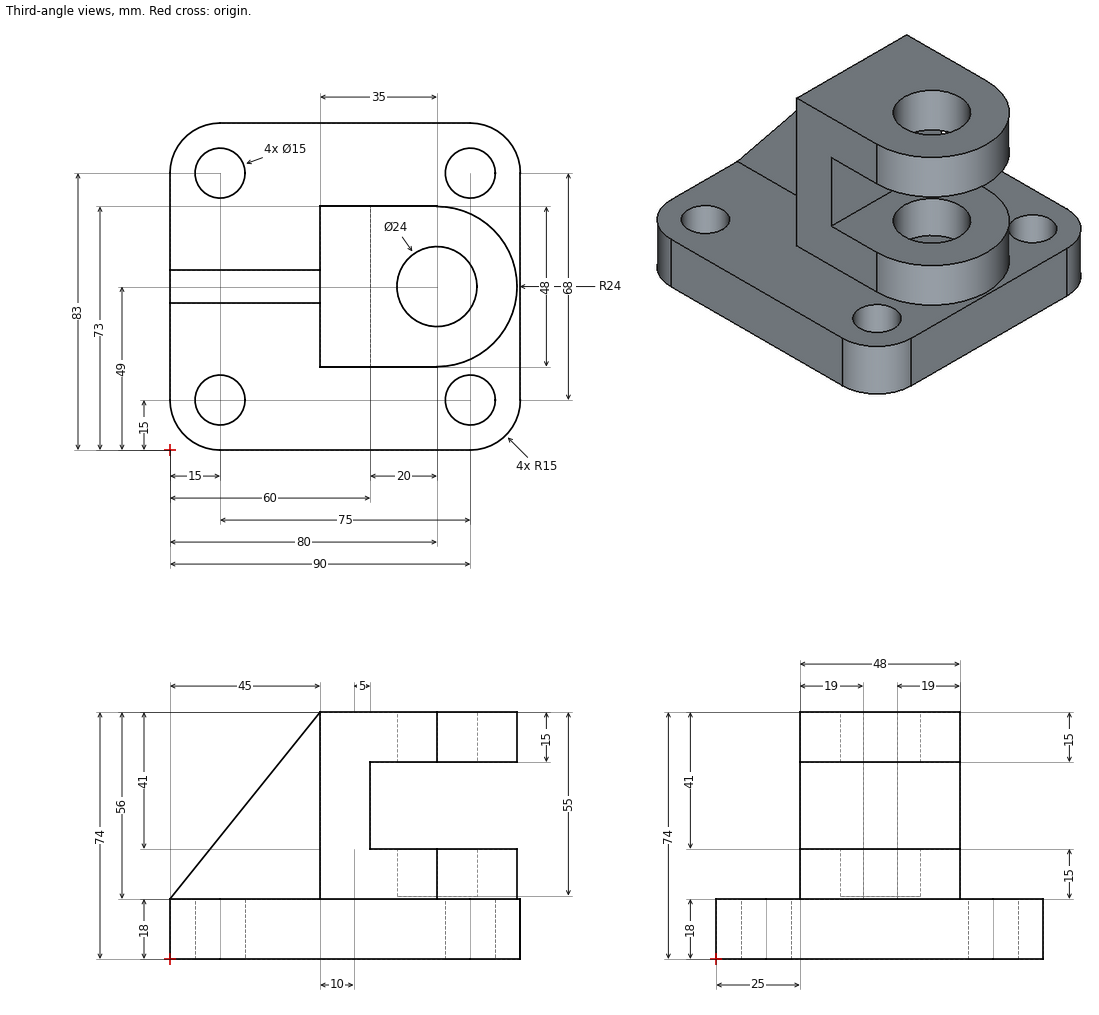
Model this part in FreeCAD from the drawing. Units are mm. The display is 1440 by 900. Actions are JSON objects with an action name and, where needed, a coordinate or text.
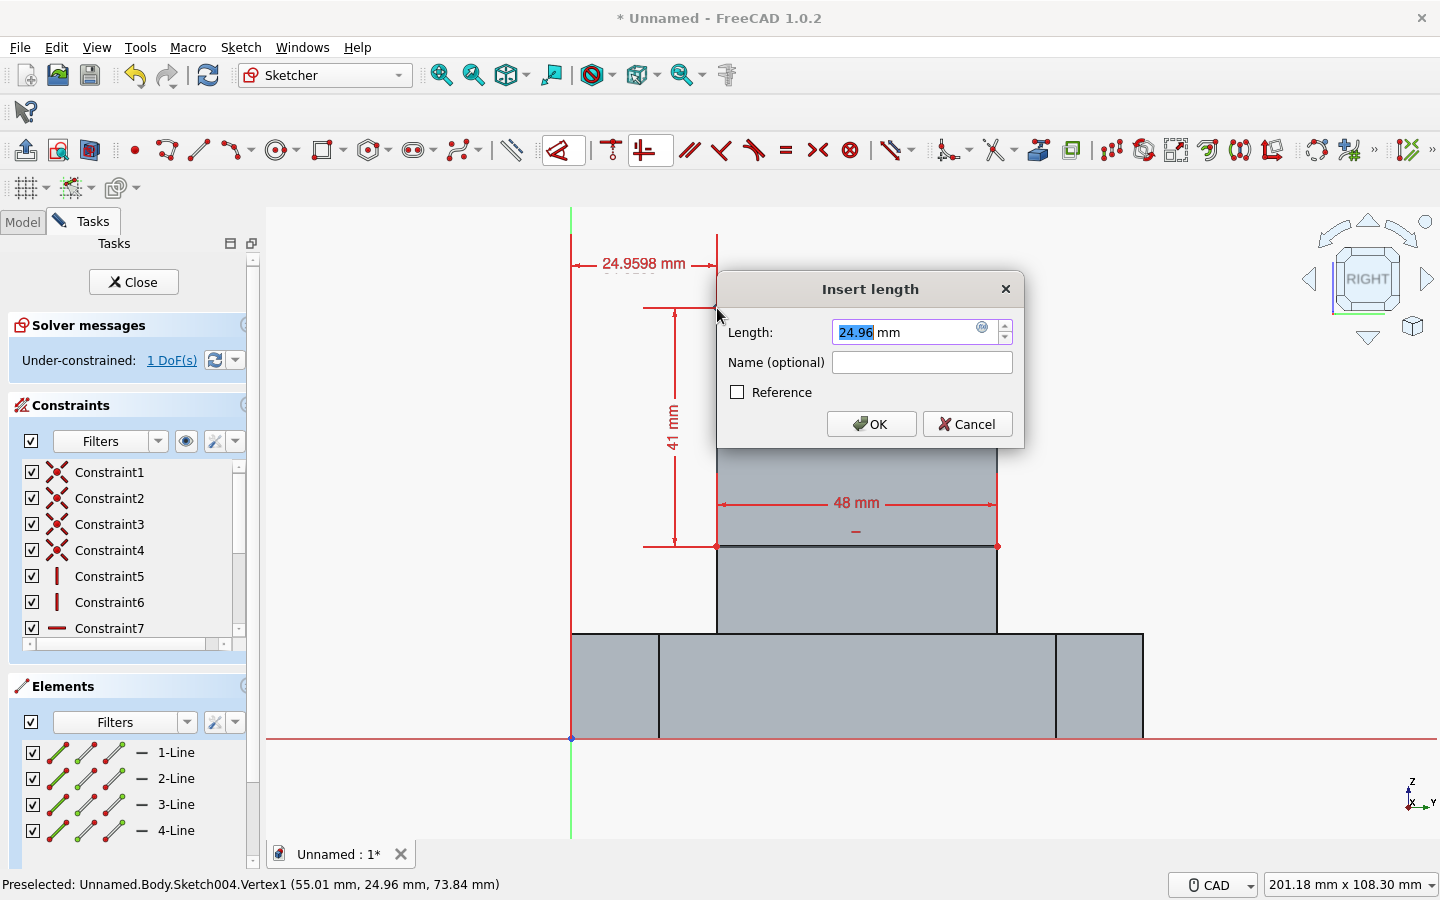
{"action": "type", "text": "25"}
{"action": "key", "text": "Return"}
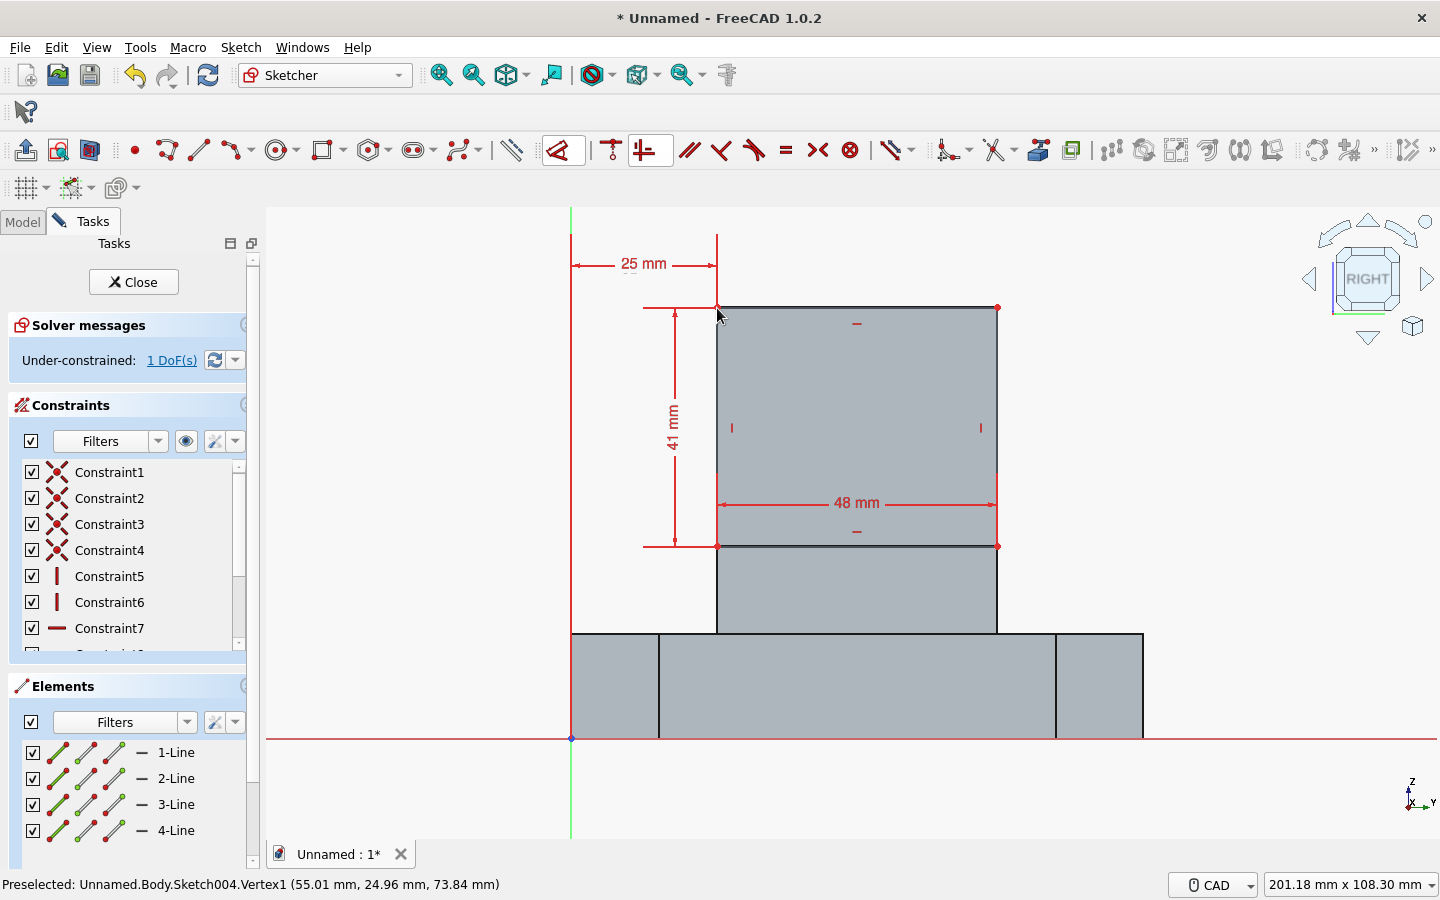
{"action": "left_click", "coordinate": [717, 308]}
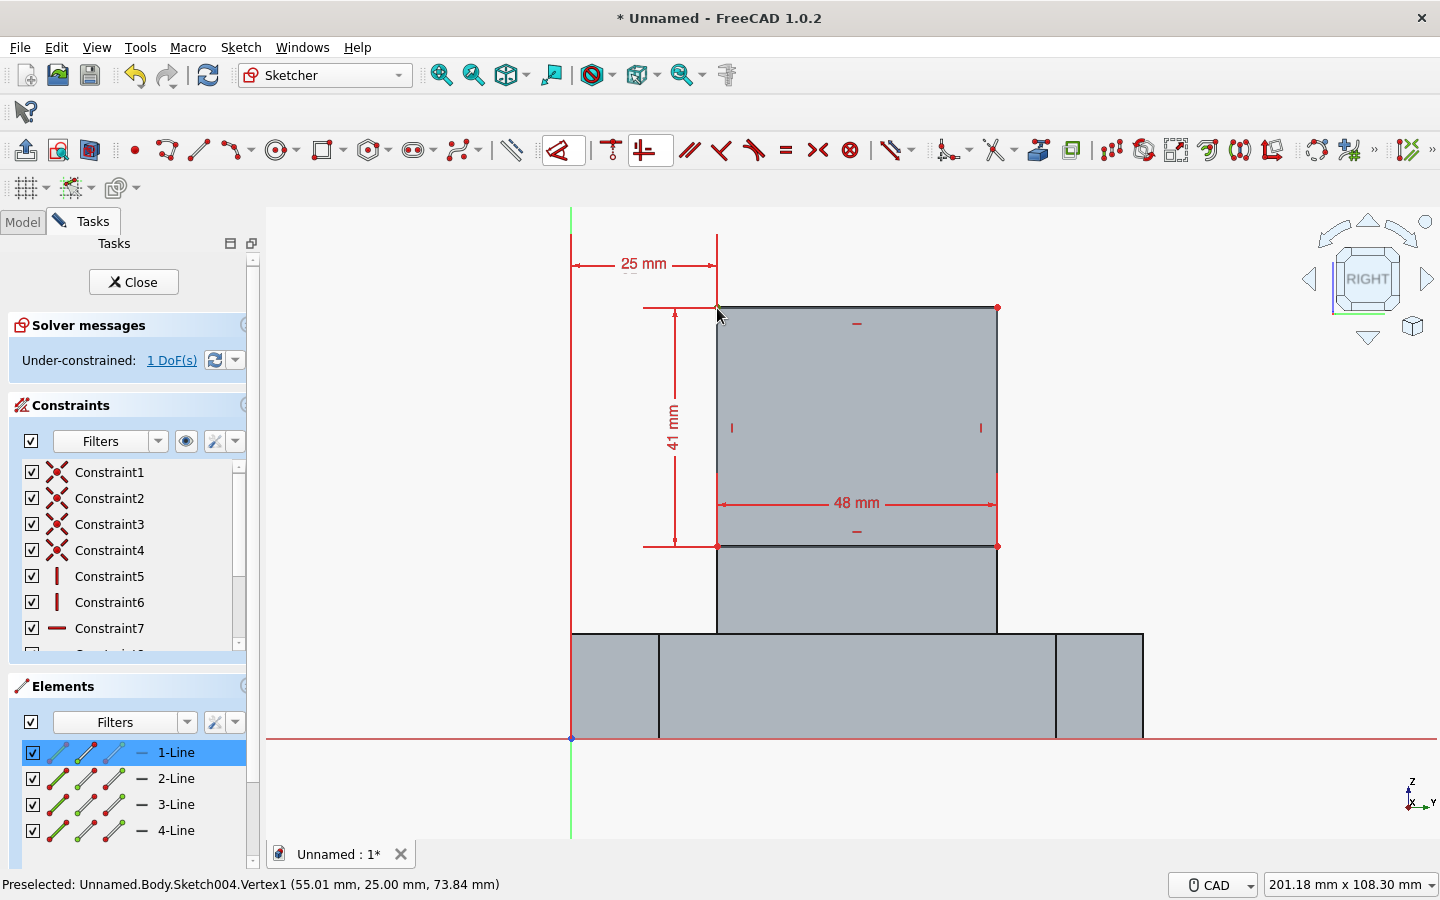
{"action": "left_click", "coordinate": [580, 150]}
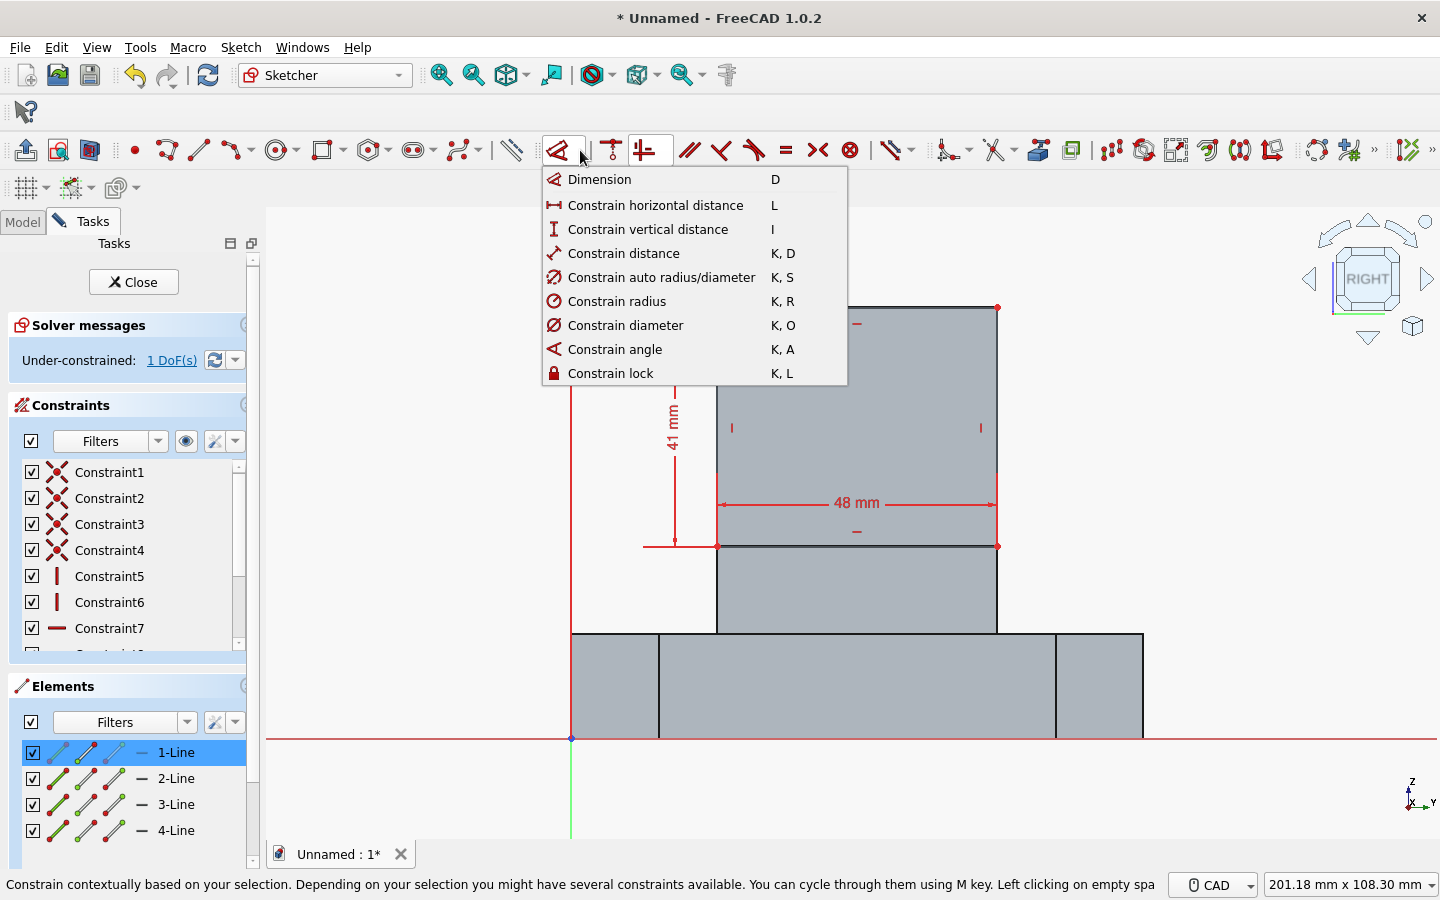
{"action": "left_click", "coordinate": [695, 229]}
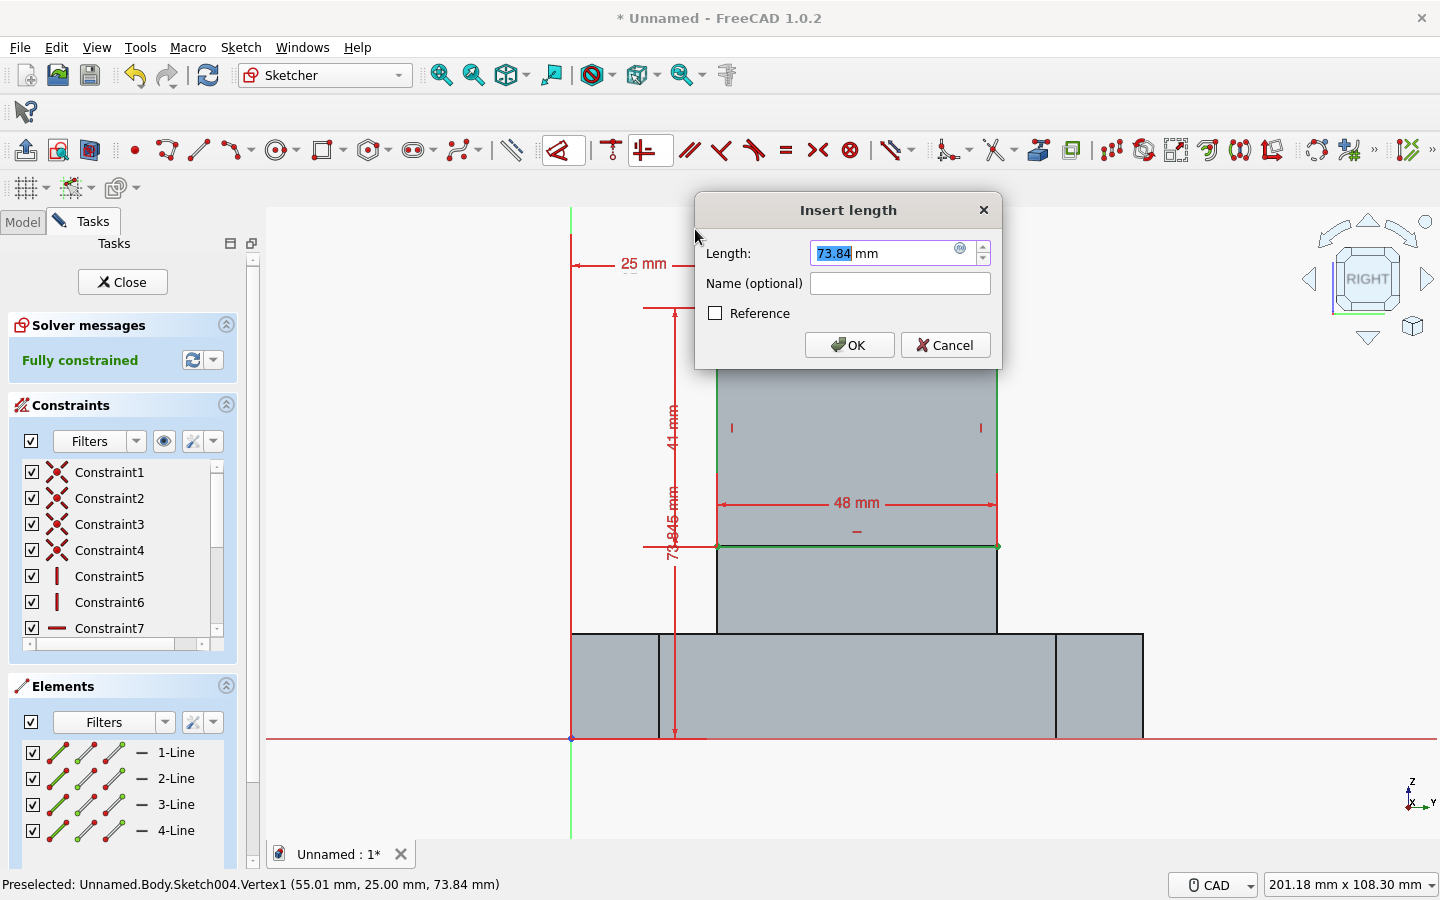
{"action": "type", "text": "74"}
{"action": "key", "text": "Return"}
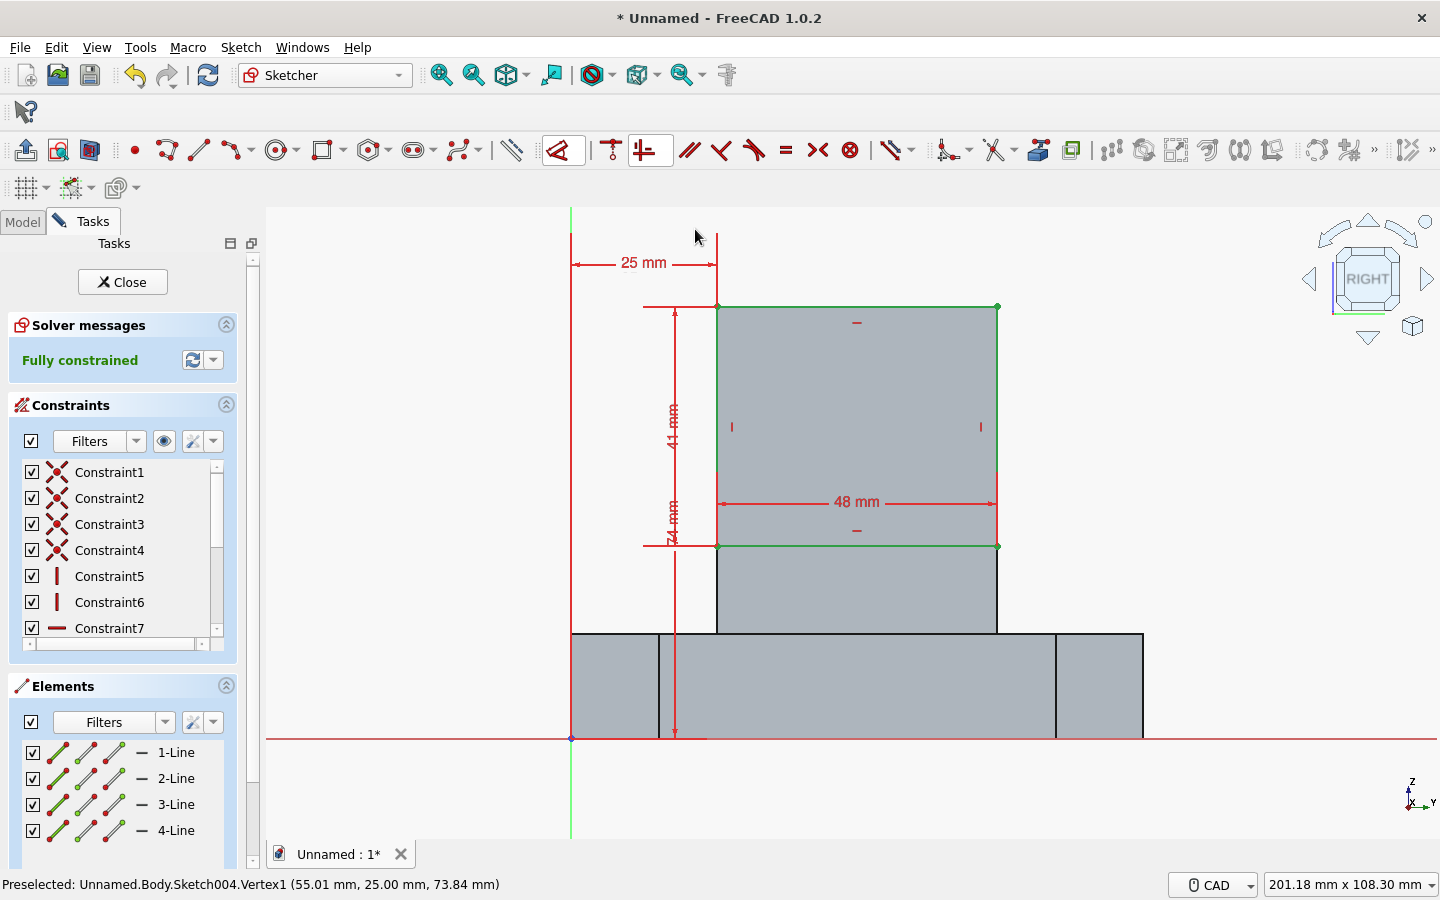
{"action": "left_click", "coordinate": [123, 282]}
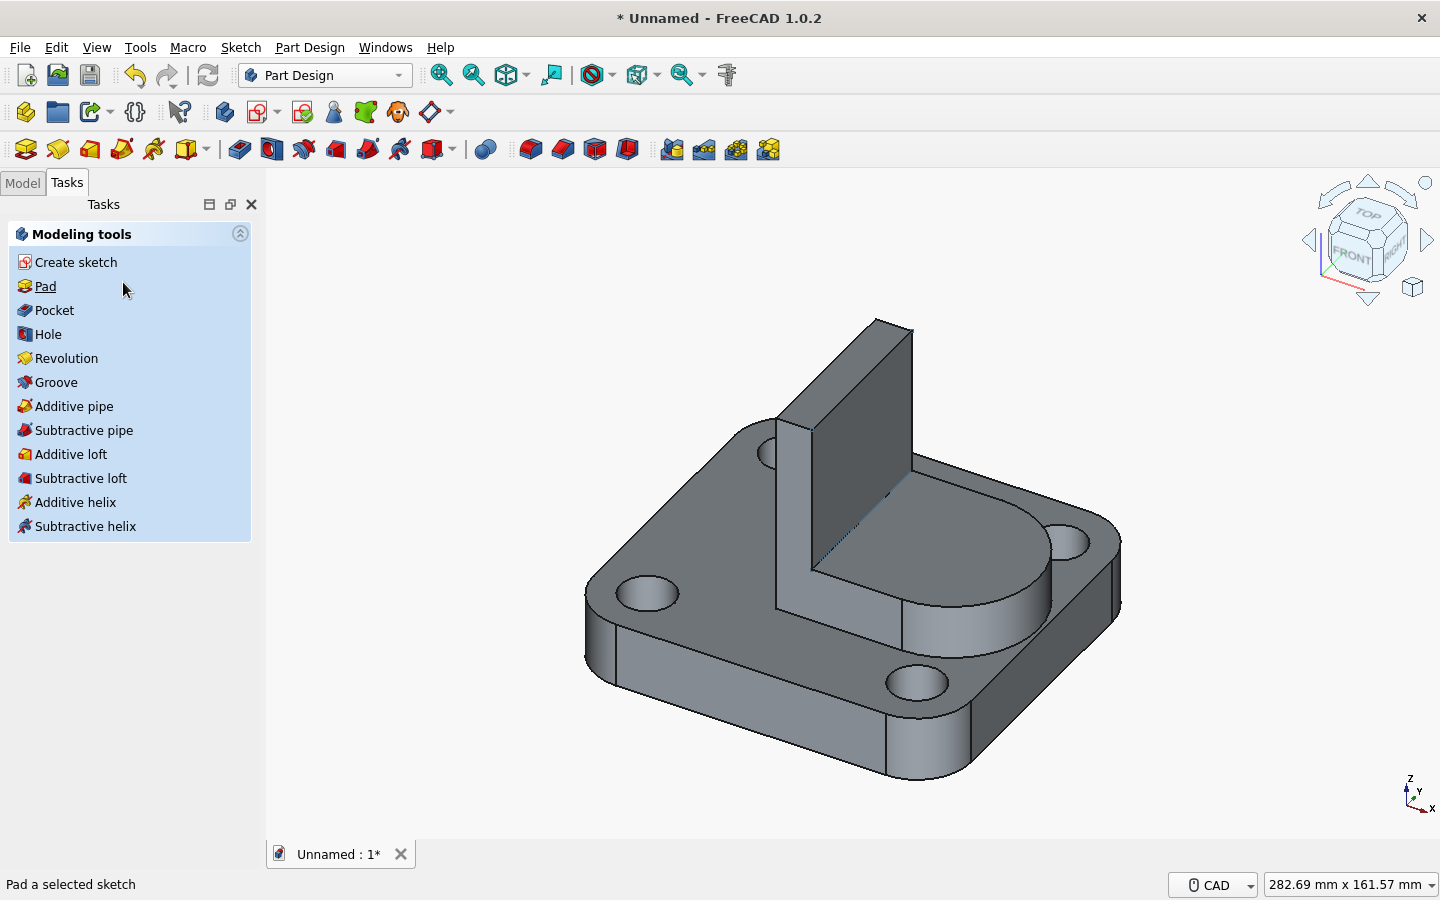
{"action": "left_click", "coordinate": [26, 150]}